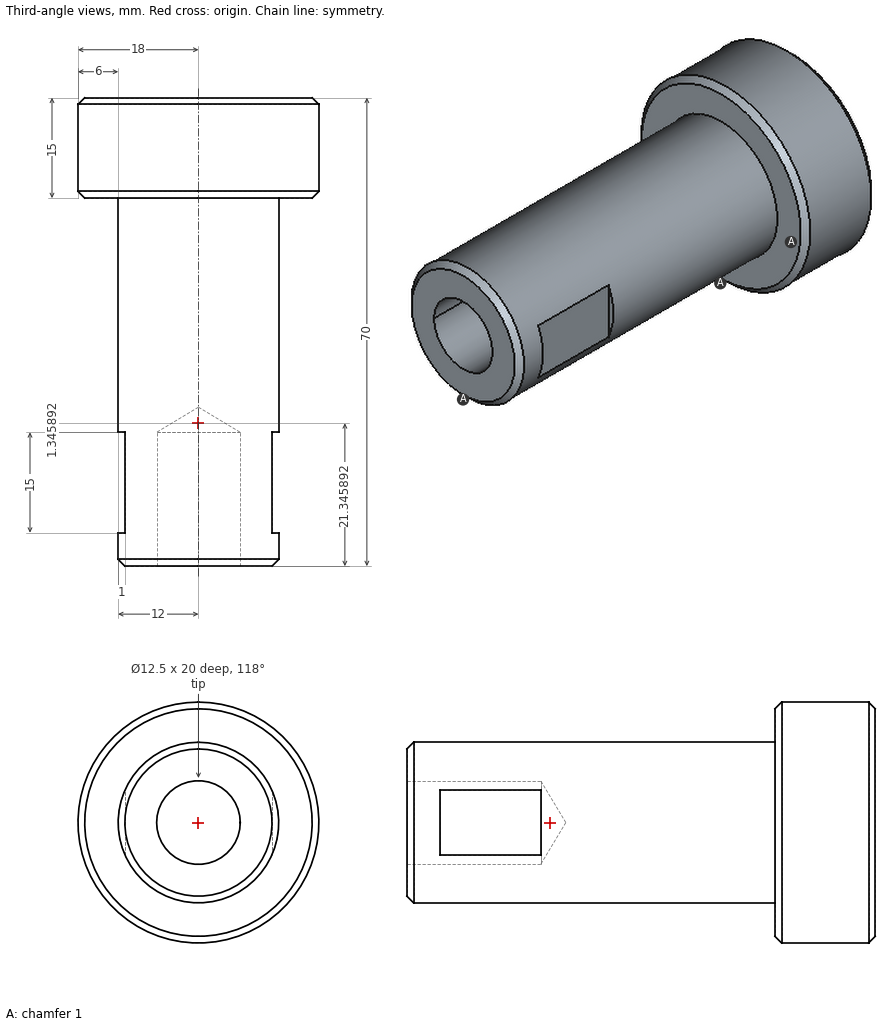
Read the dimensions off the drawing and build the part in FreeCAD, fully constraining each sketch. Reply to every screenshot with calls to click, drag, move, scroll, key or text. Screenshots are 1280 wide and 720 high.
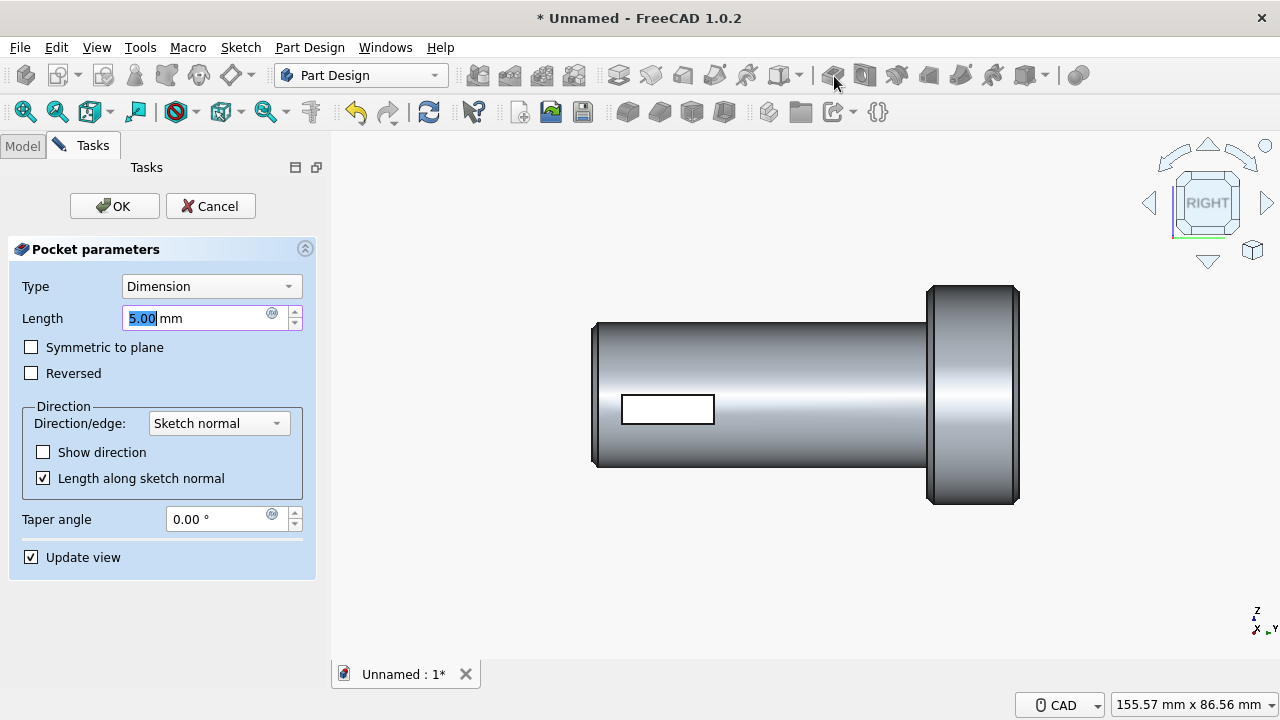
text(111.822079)
key(Tab)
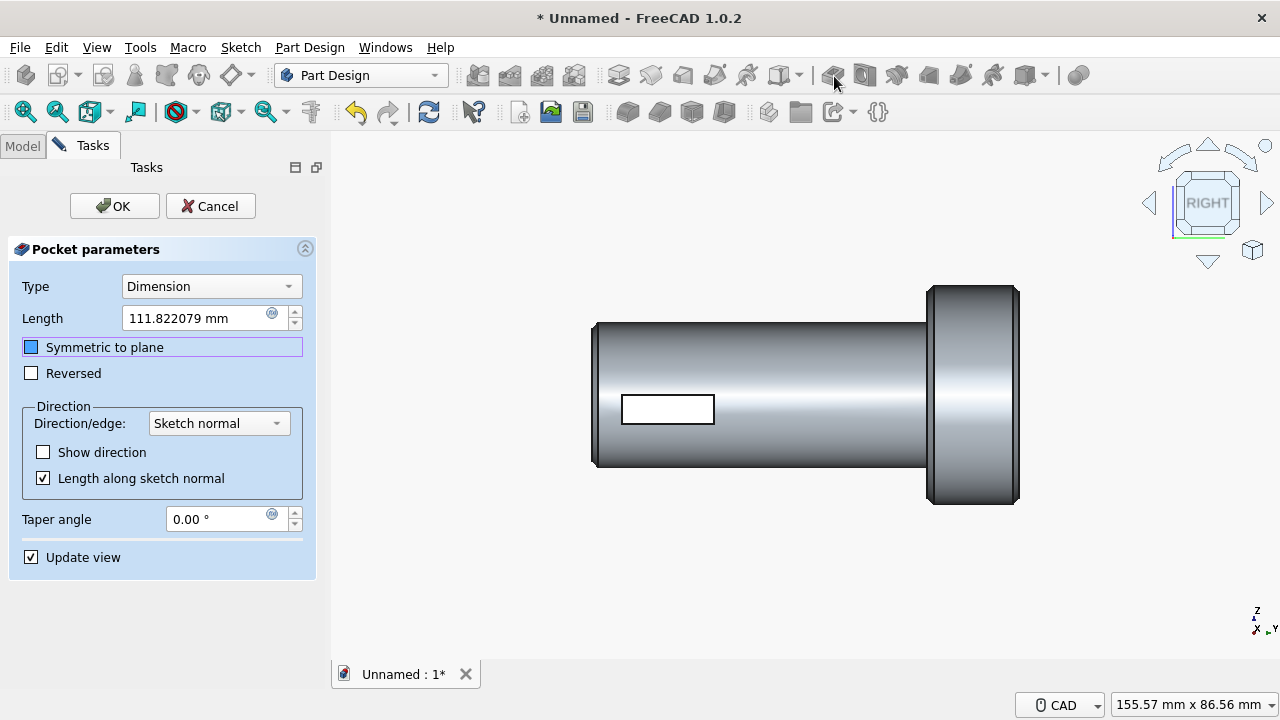
click(30, 347)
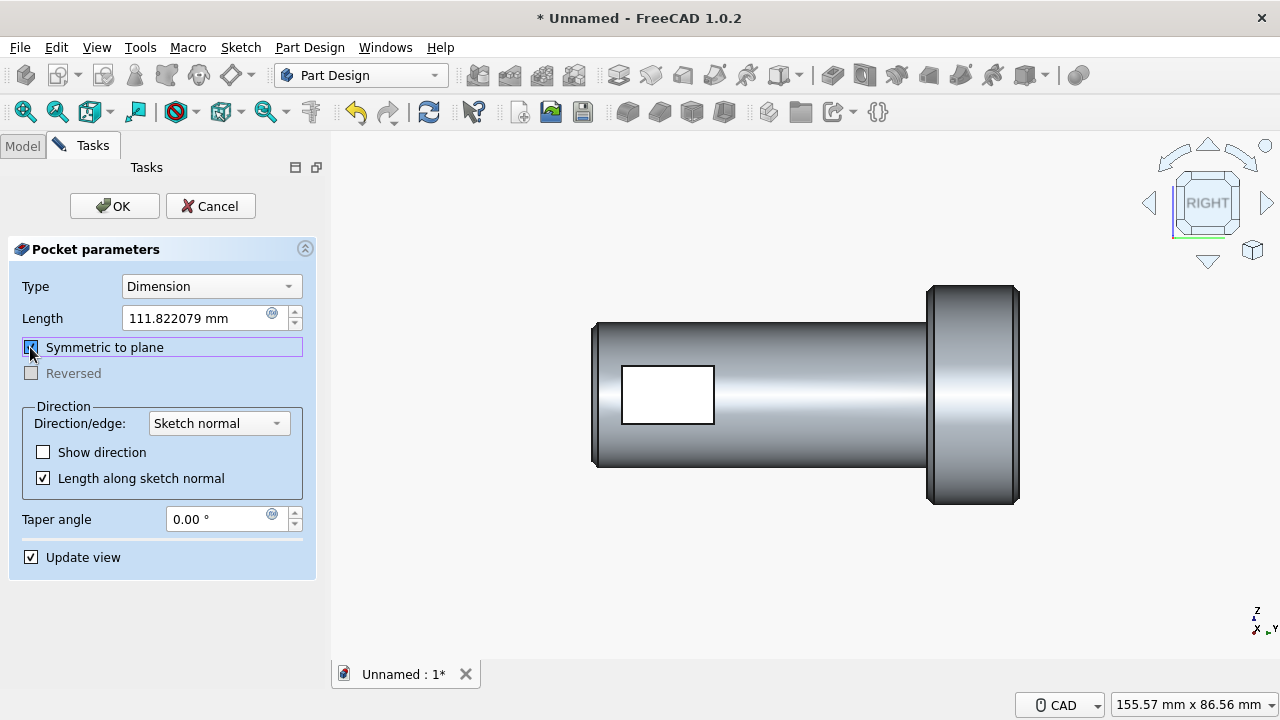
click(115, 206)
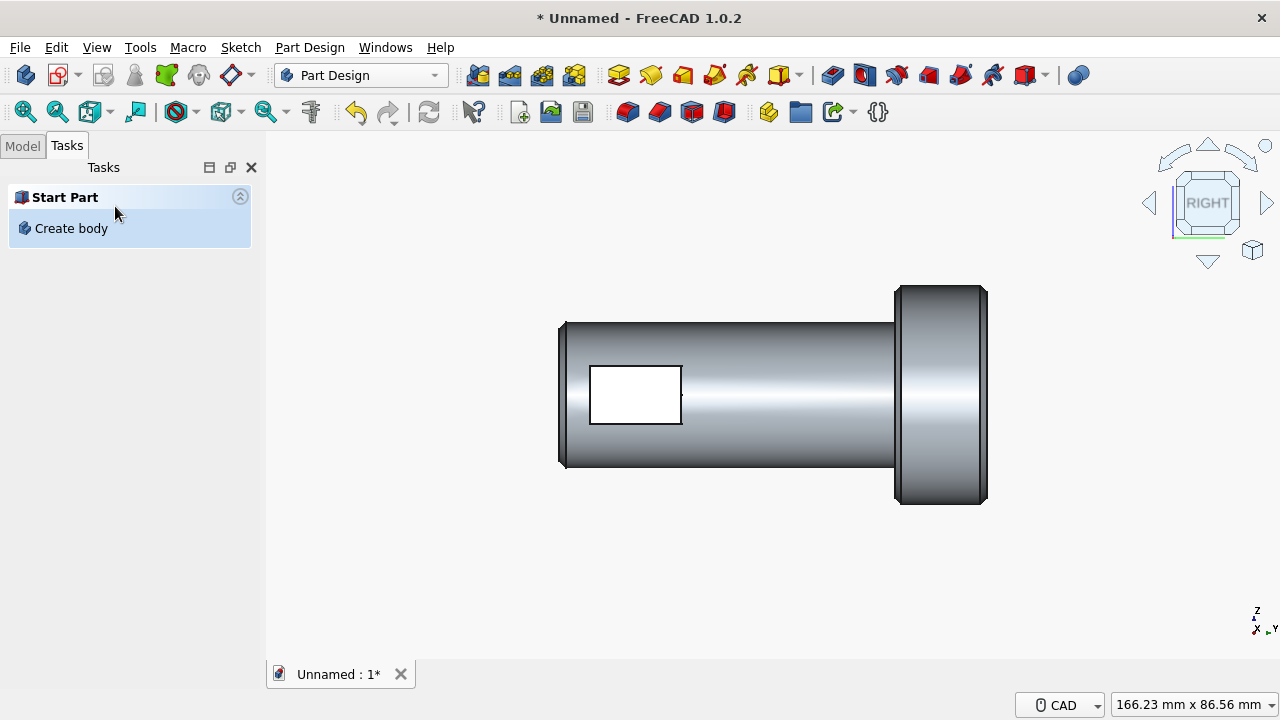
click(26, 112)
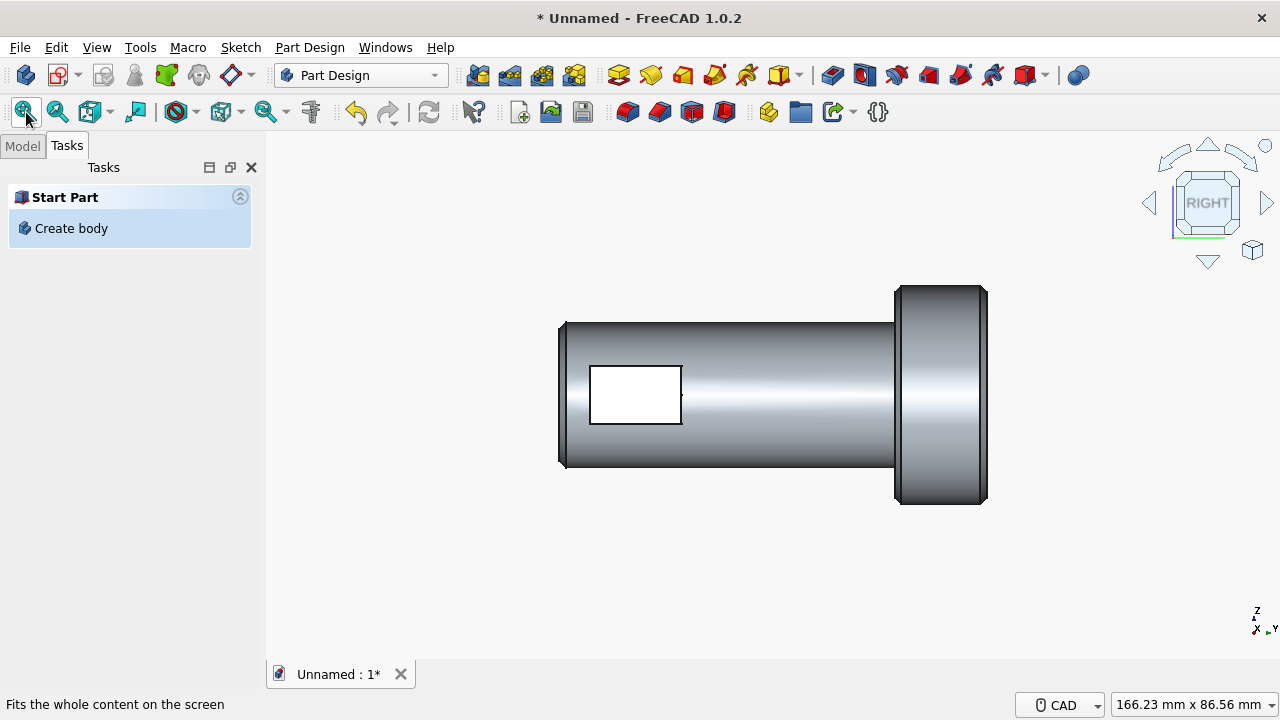
key(0)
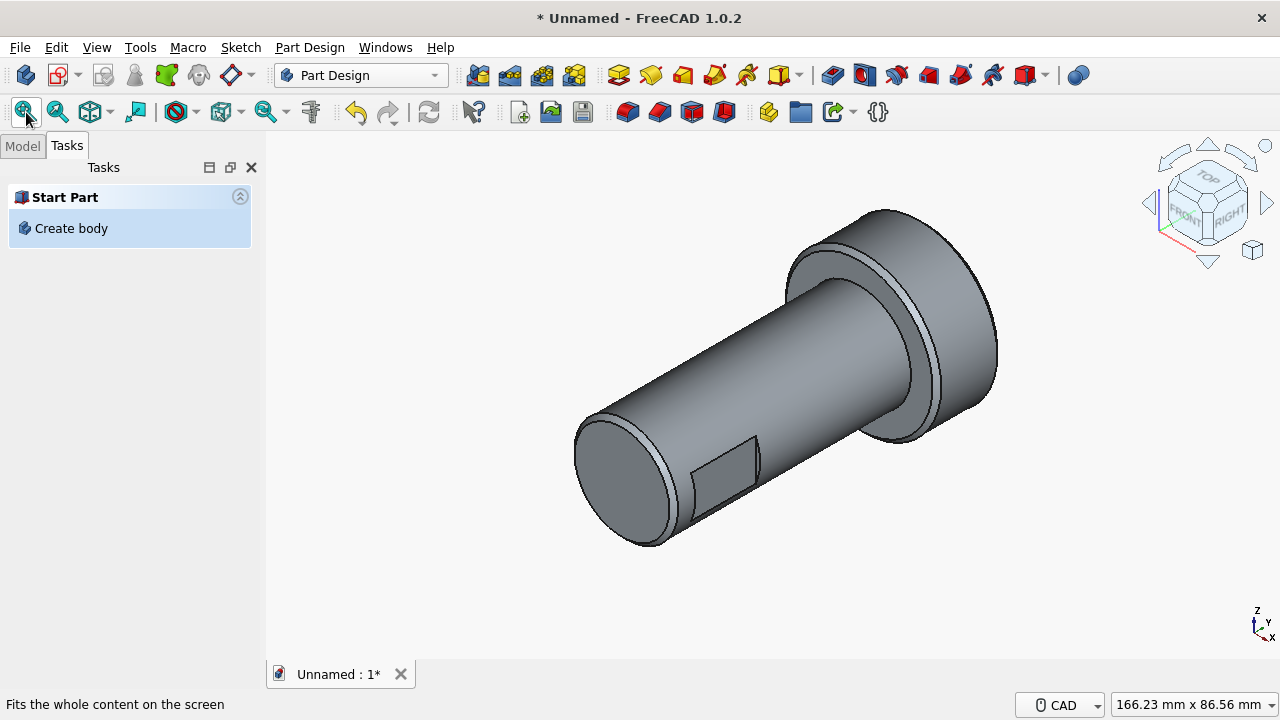
click(622, 481)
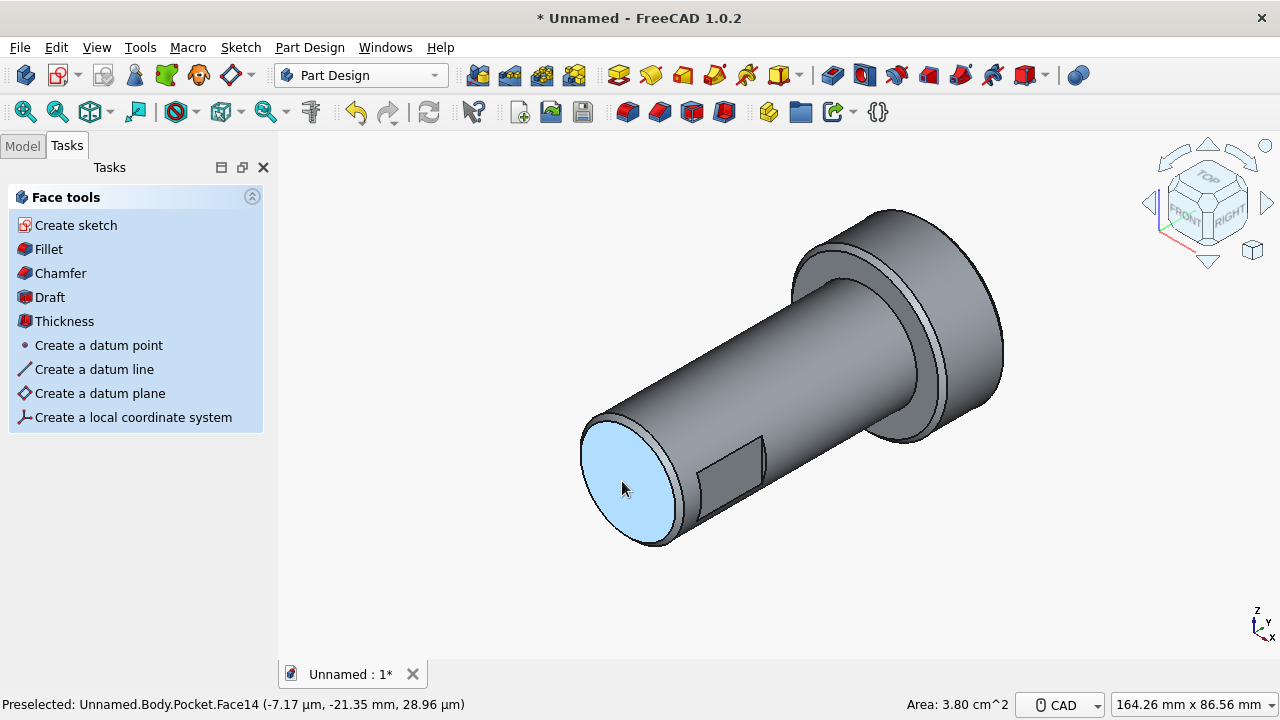
click(58, 76)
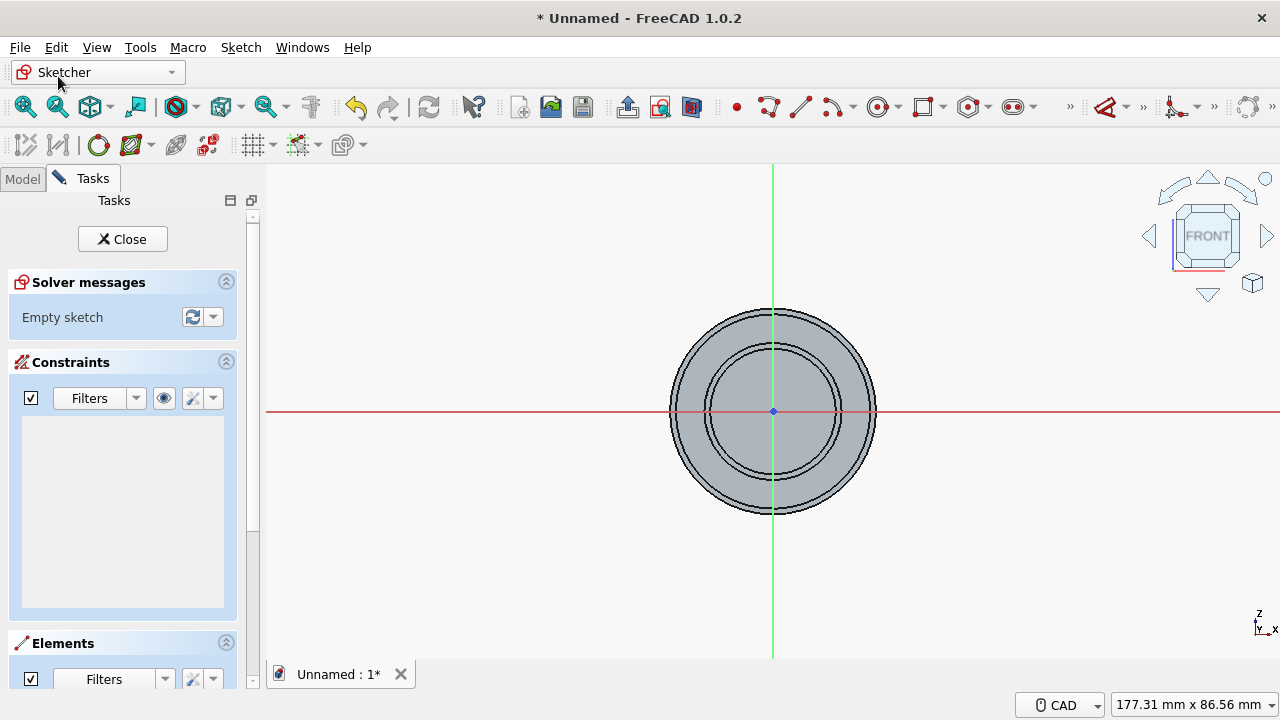
scroll(795, 412, up, 7)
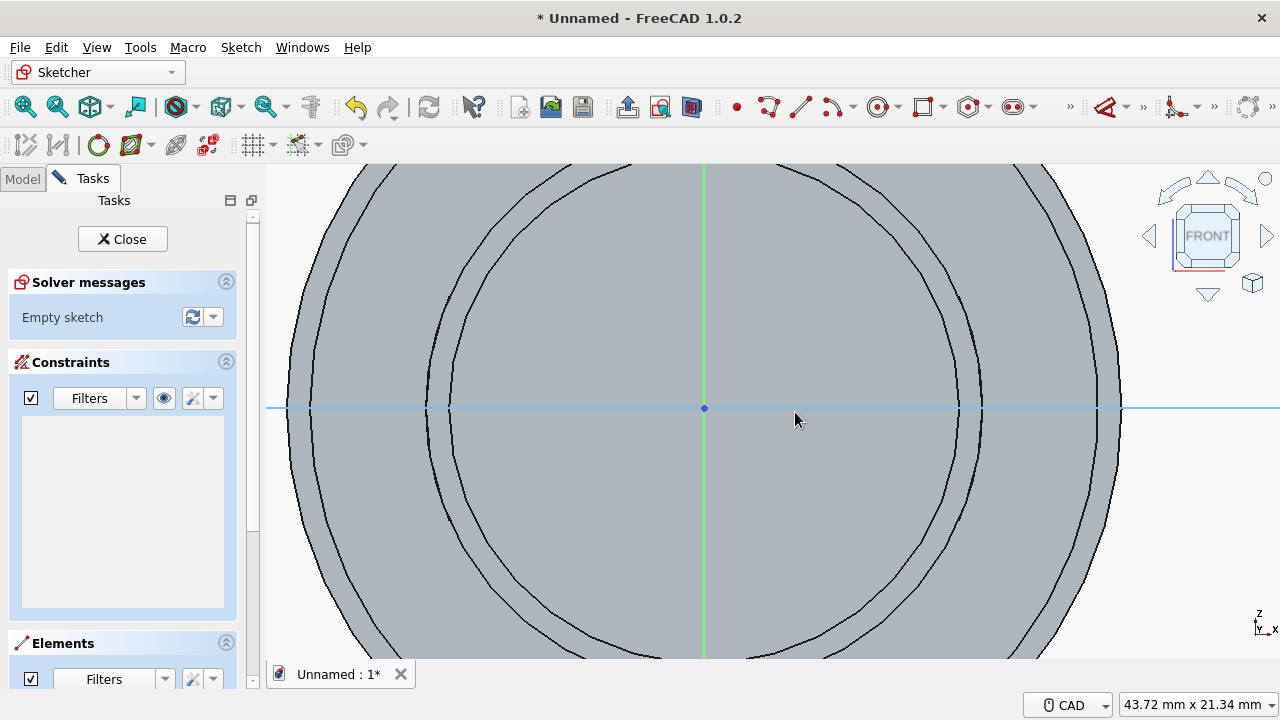
click(878, 108)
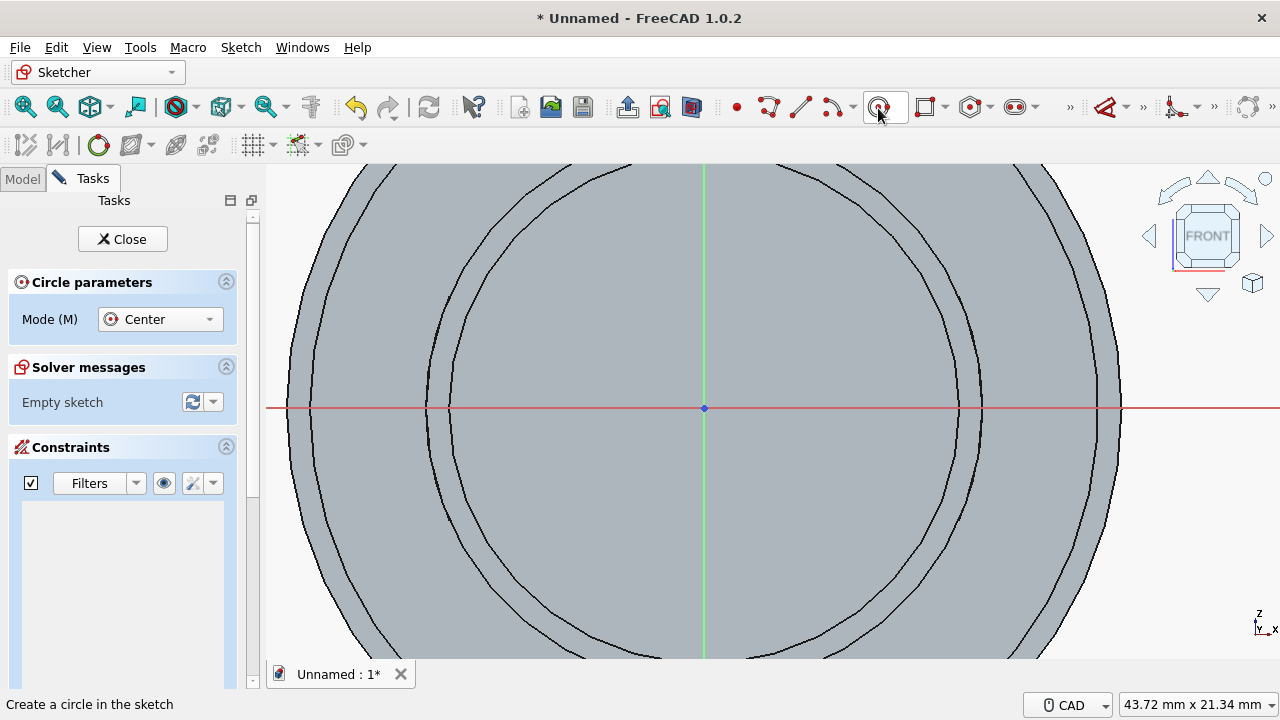
click(704, 408)
click(807, 306)
key(Escape)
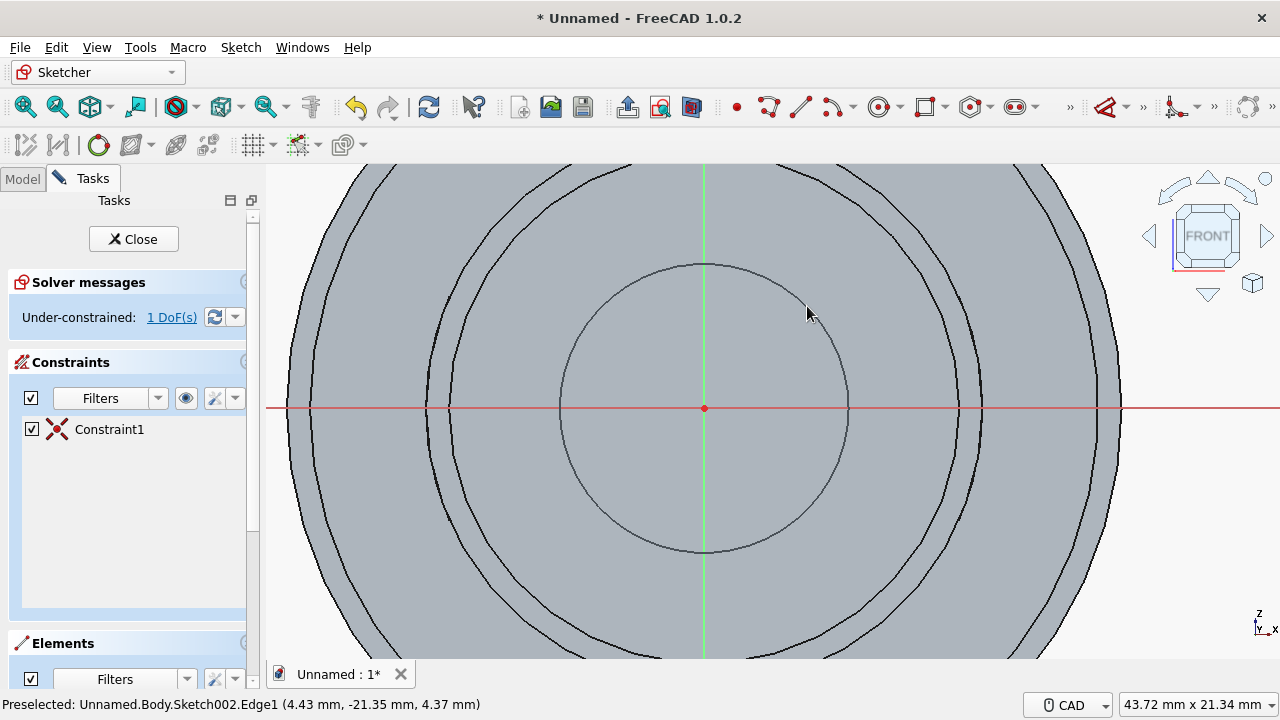
click(1106, 108)